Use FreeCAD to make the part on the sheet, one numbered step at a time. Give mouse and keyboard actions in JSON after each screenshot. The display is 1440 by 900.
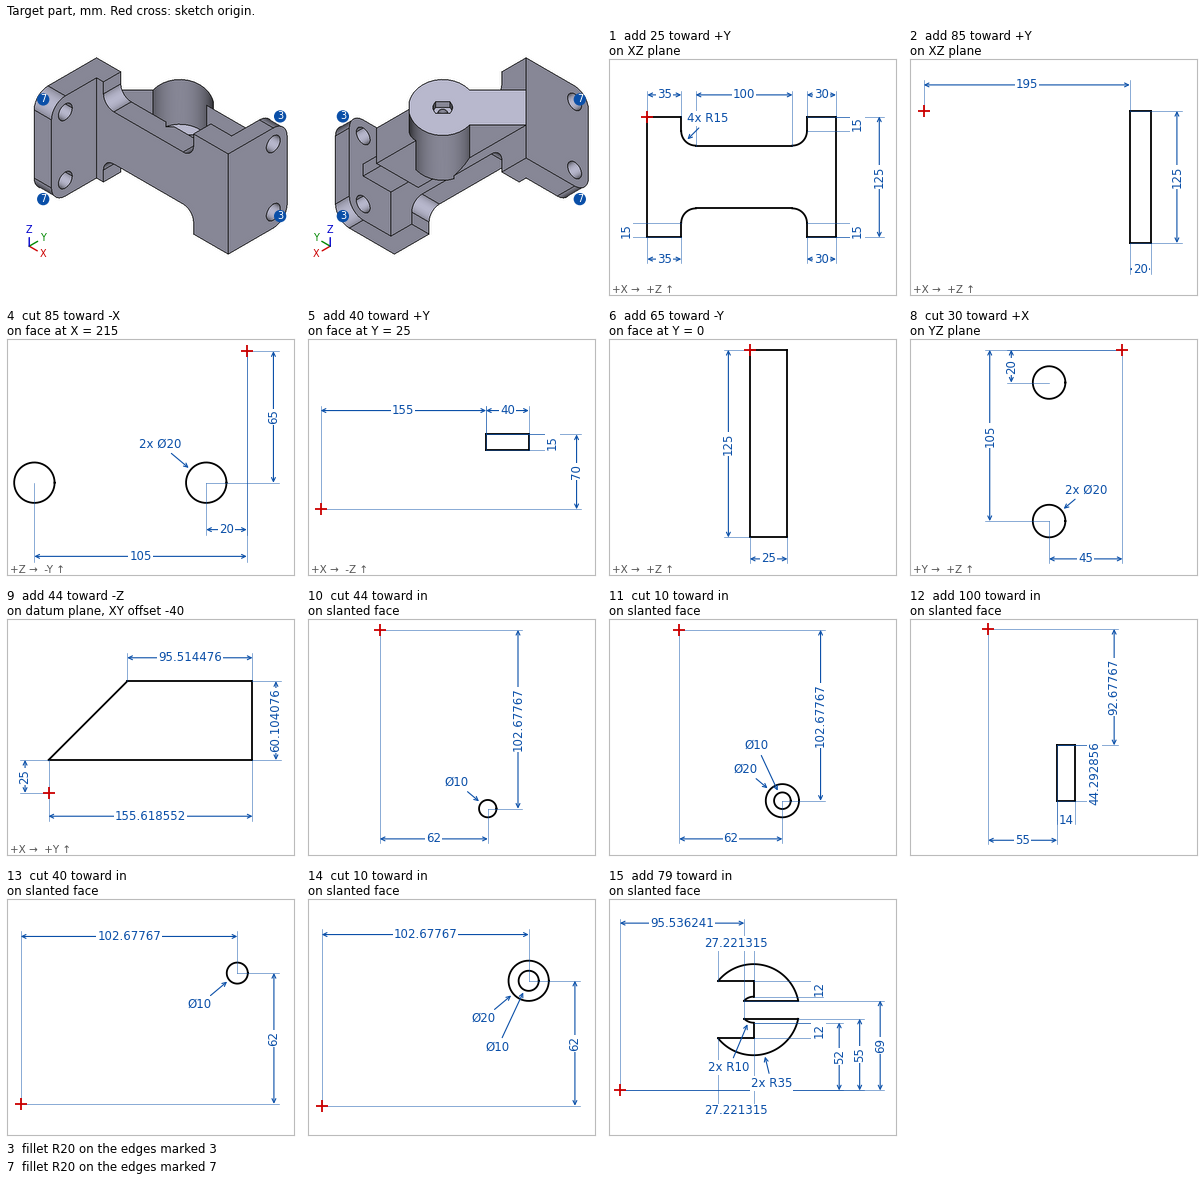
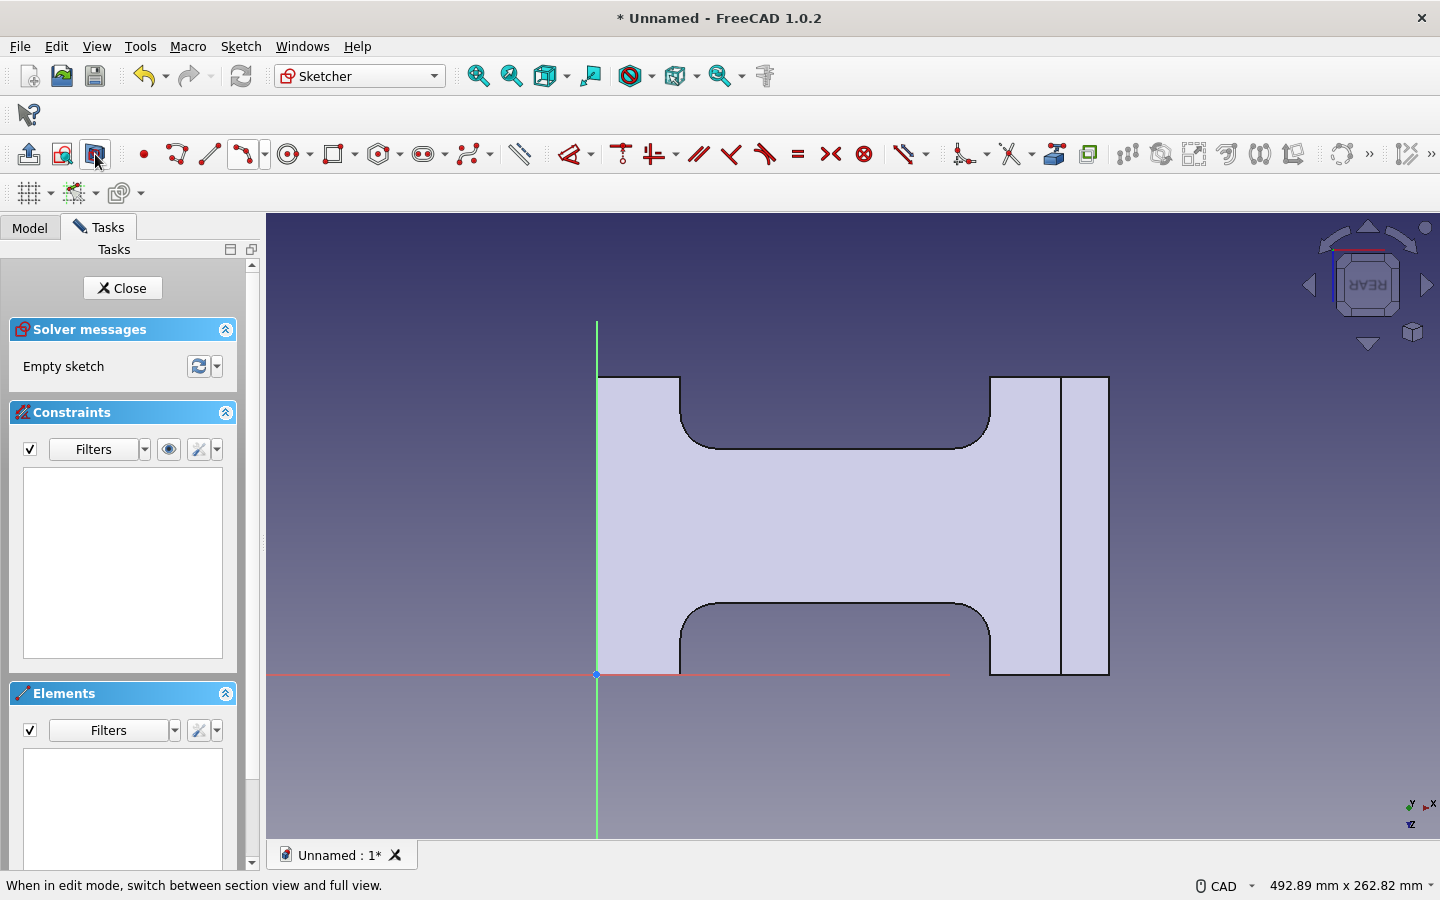
{"action": "scroll", "coordinate": [1050, 526], "scroll_direction": "up", "scroll_amount": 10}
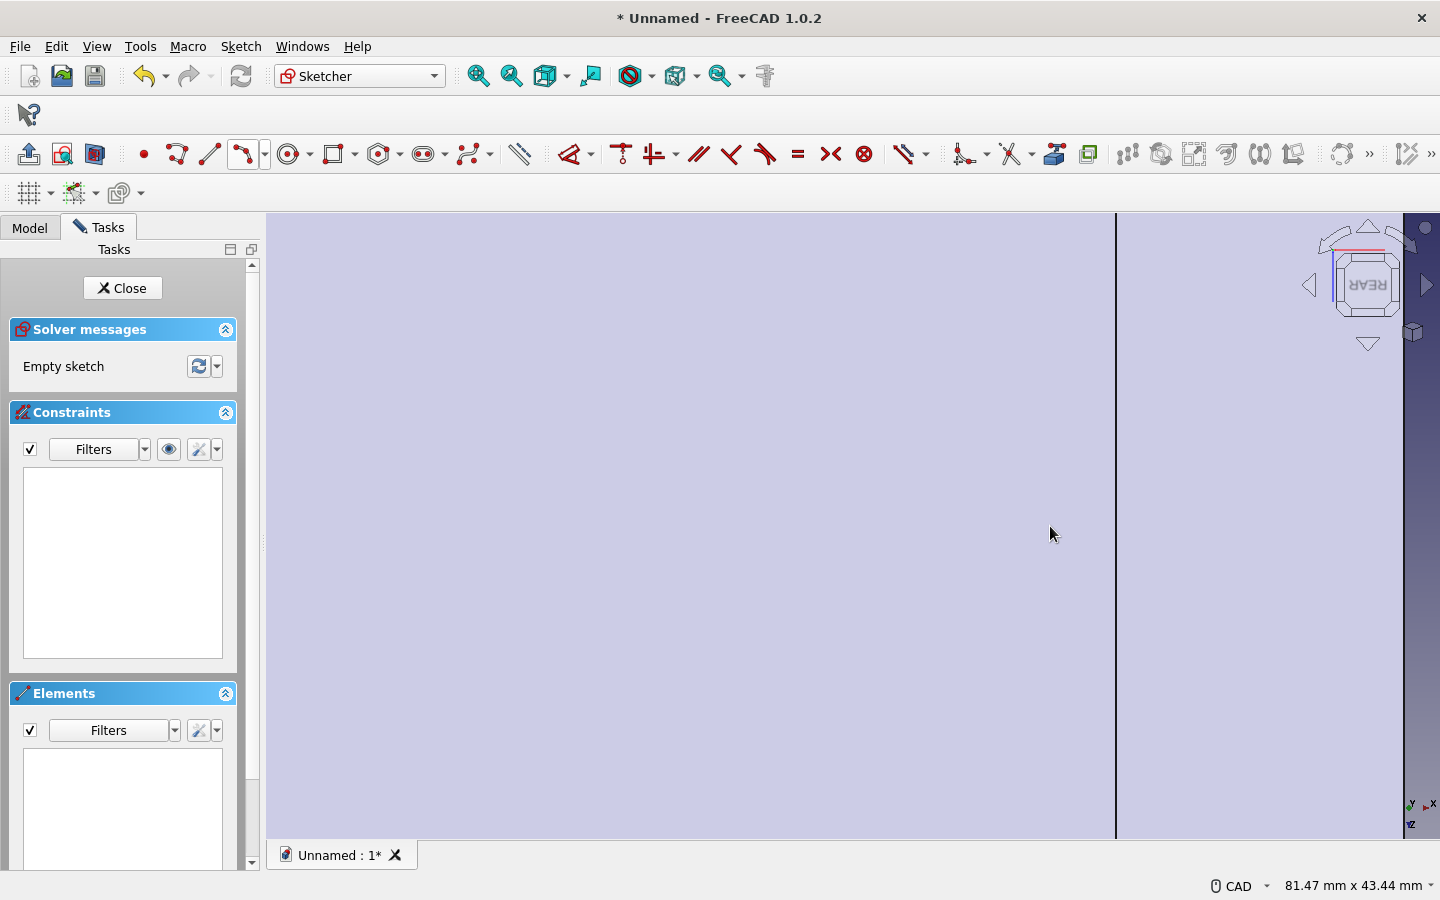
{"action": "left_click", "coordinate": [332, 154]}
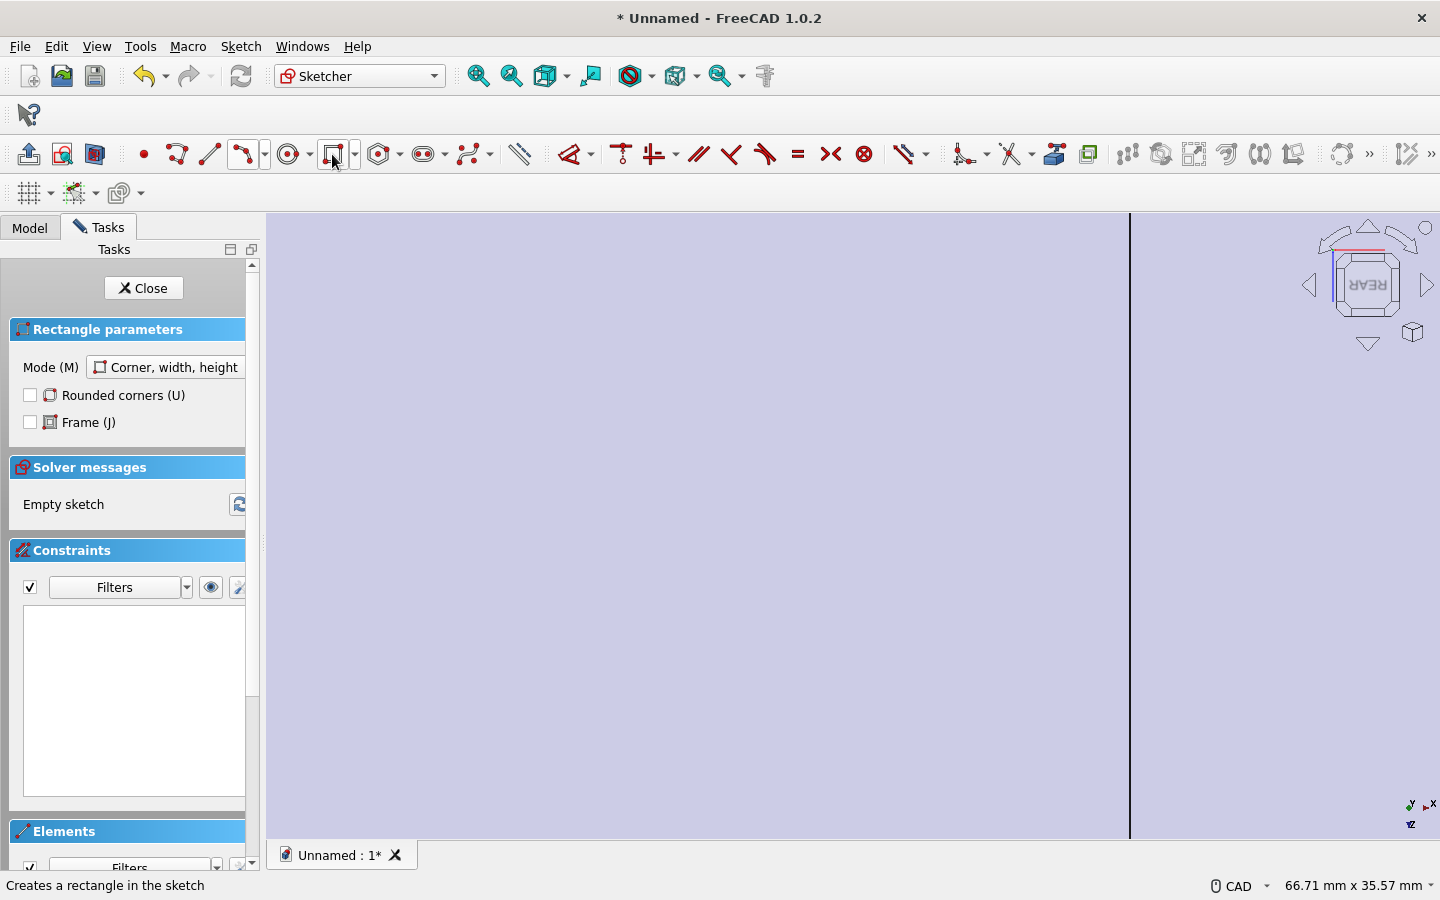
{"action": "left_click", "coordinate": [426, 391]}
{"action": "left_click", "coordinate": [1130, 655]}
{"action": "key", "text": "Escape"}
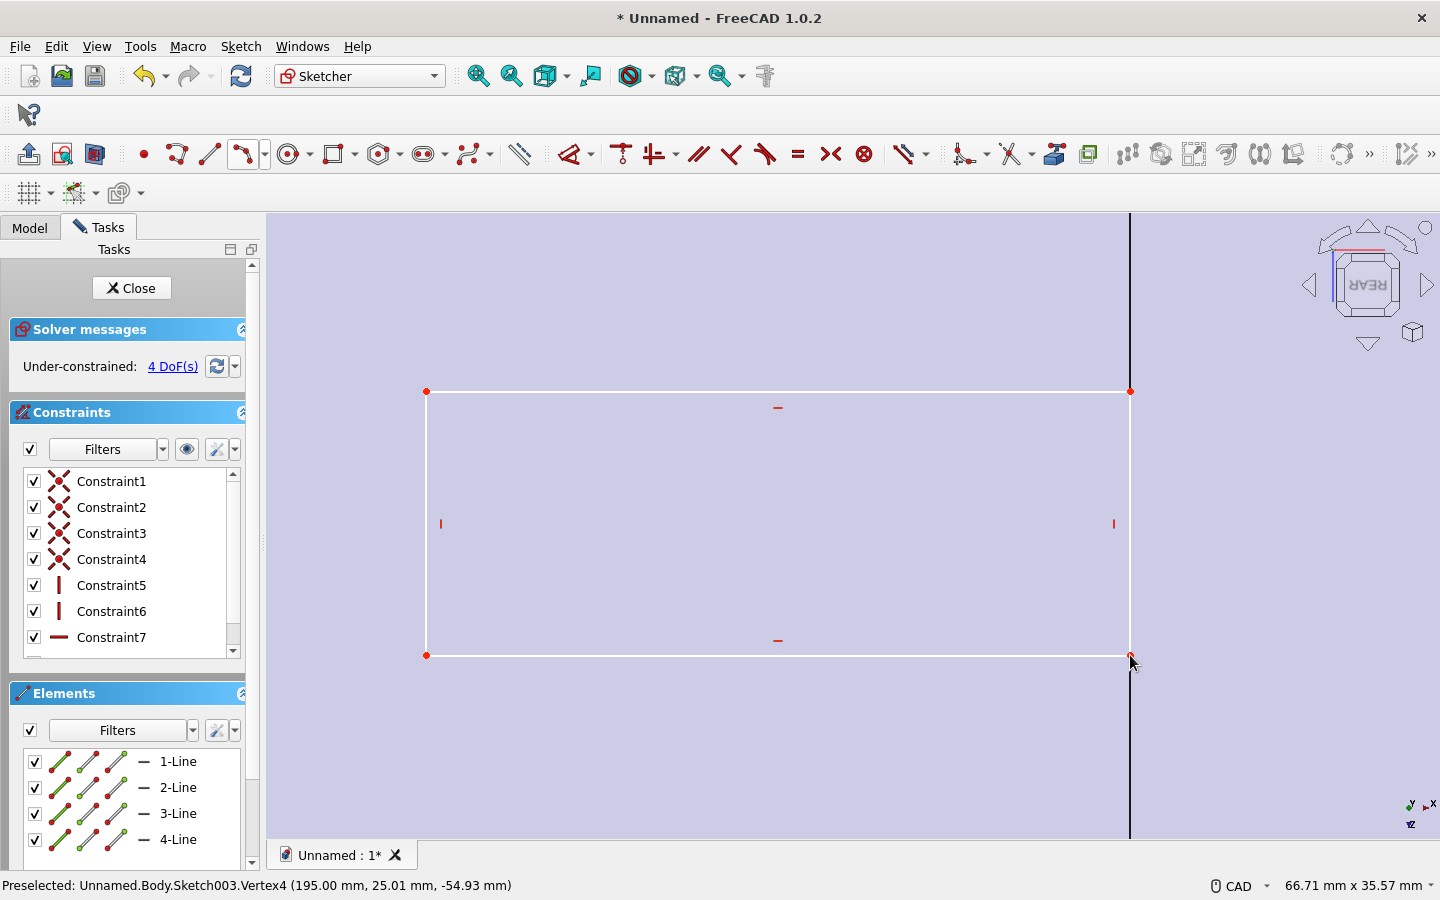
{"action": "left_click", "coordinate": [568, 154]}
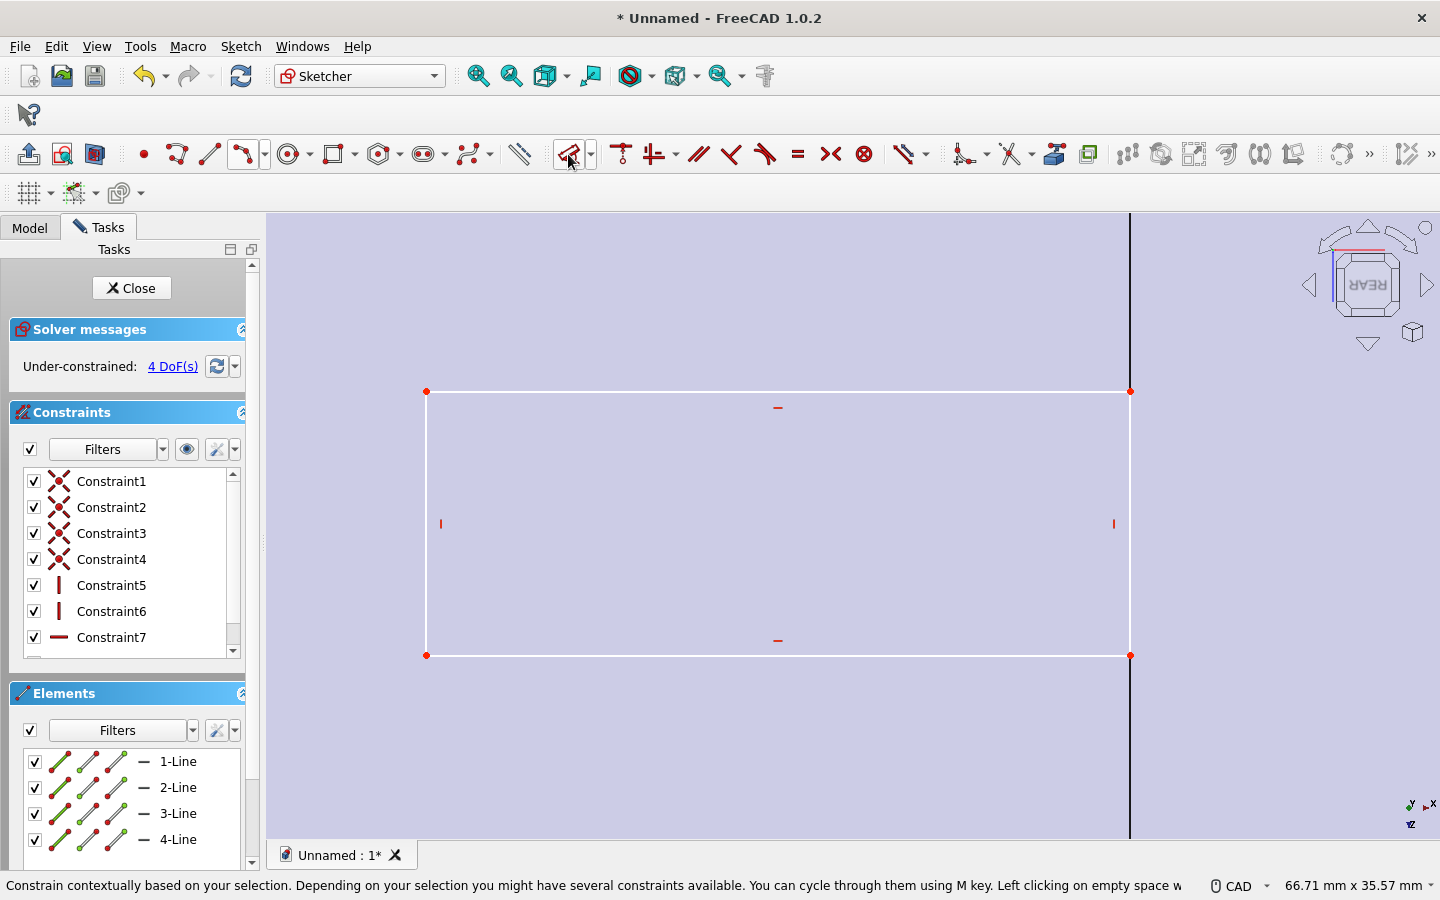
{"action": "left_click", "coordinate": [426, 471]}
{"action": "left_click", "coordinate": [392, 524]}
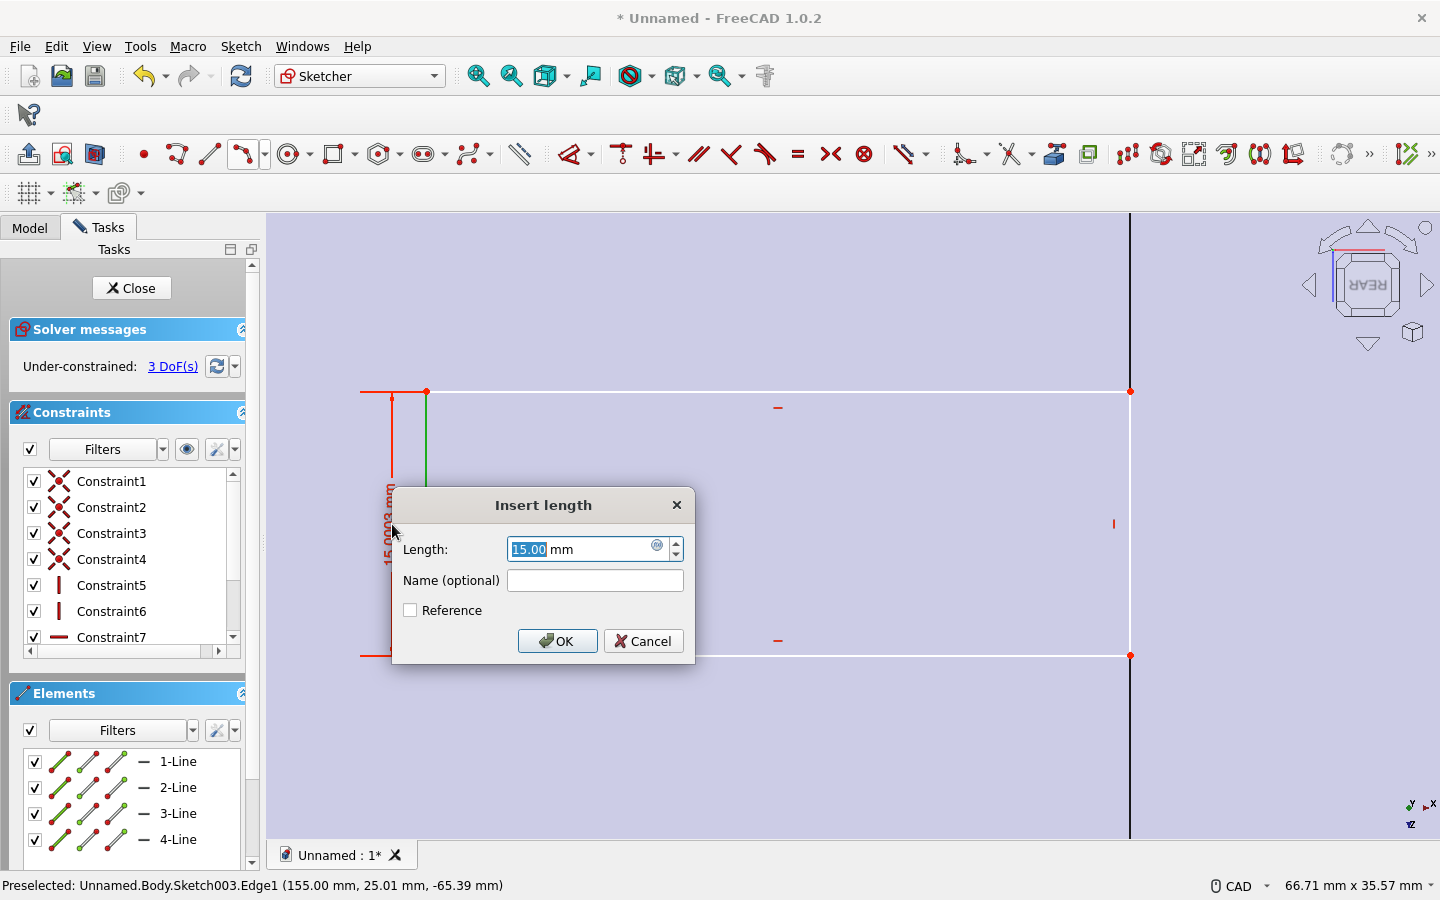
{"action": "type", "text": "15"}
{"action": "key", "text": "Return"}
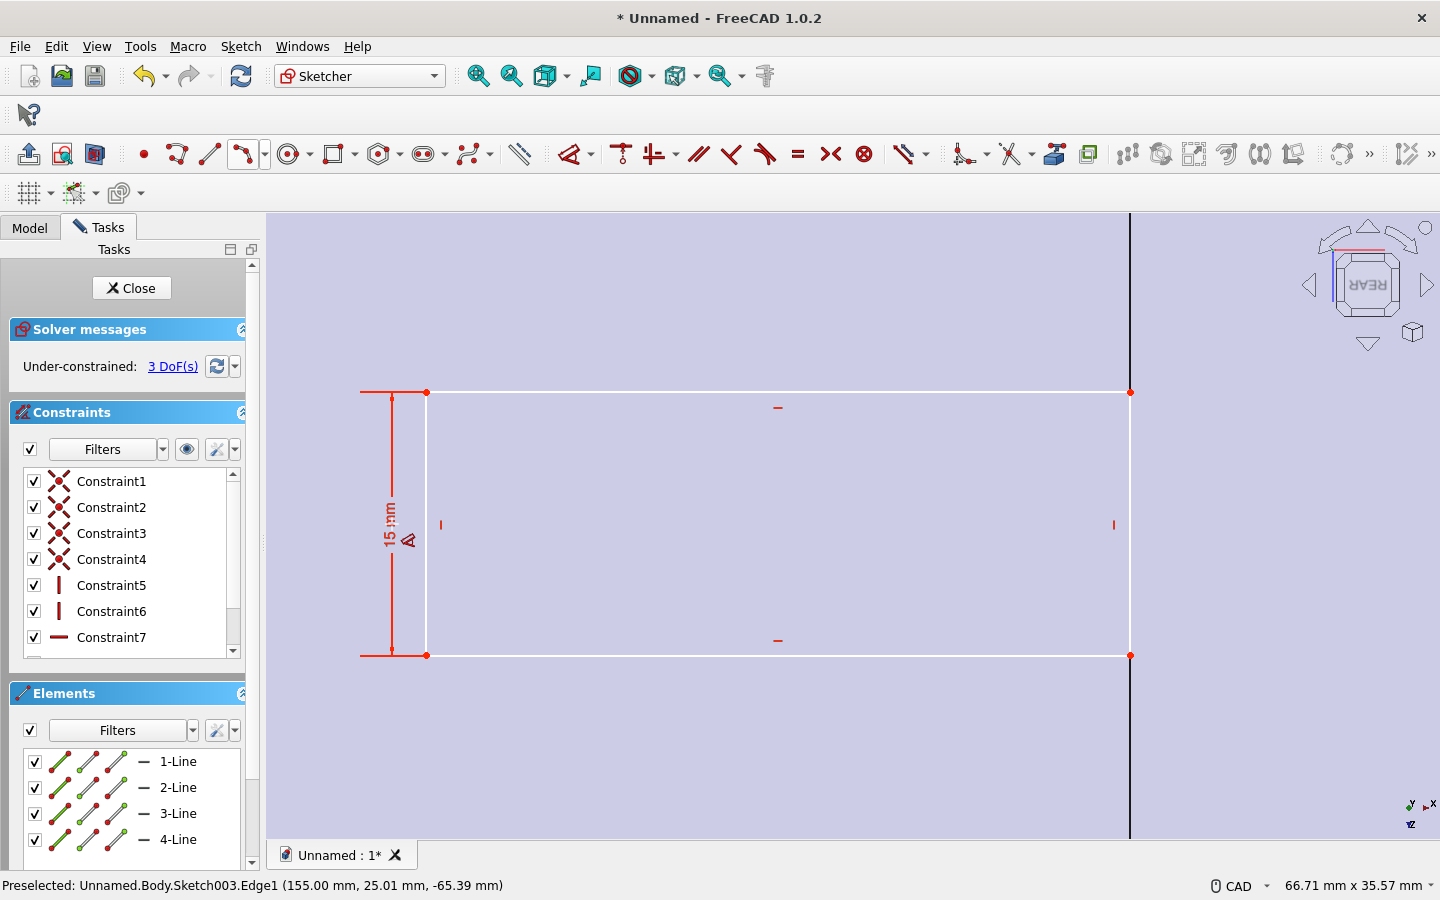
{"action": "left_click", "coordinate": [637, 656]}
{"action": "left_click", "coordinate": [778, 690]}